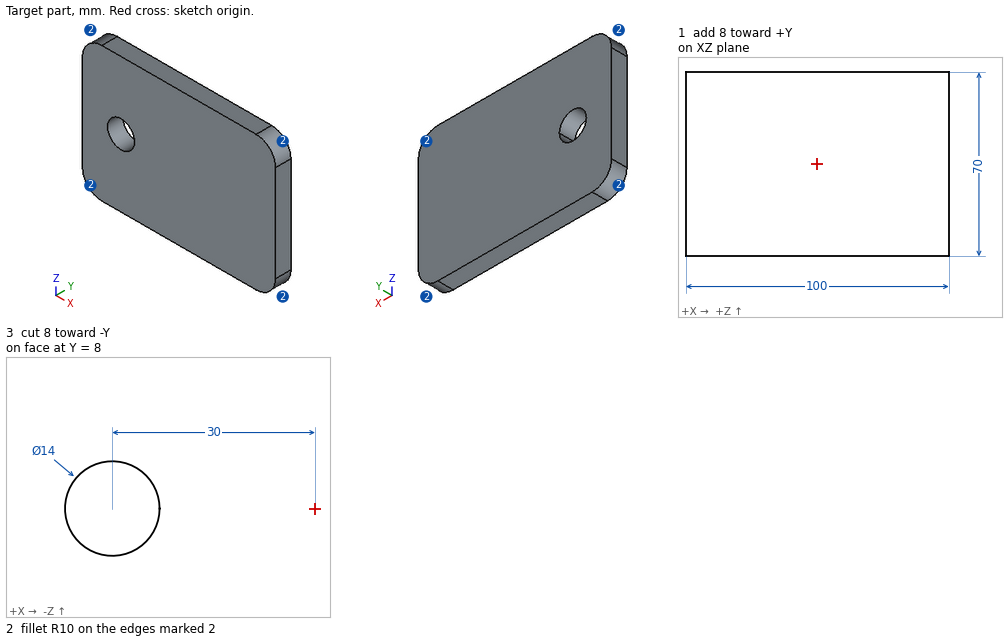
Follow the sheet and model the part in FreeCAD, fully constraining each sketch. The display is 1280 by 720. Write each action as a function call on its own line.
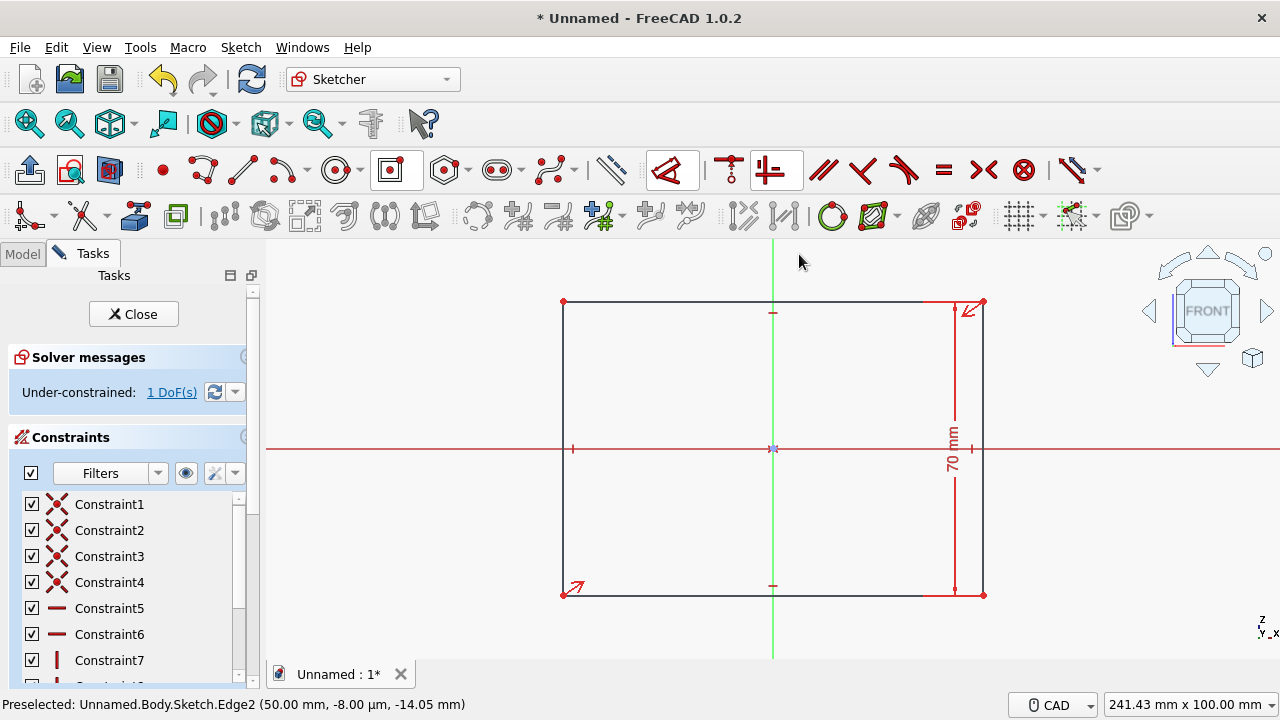
click(689, 596)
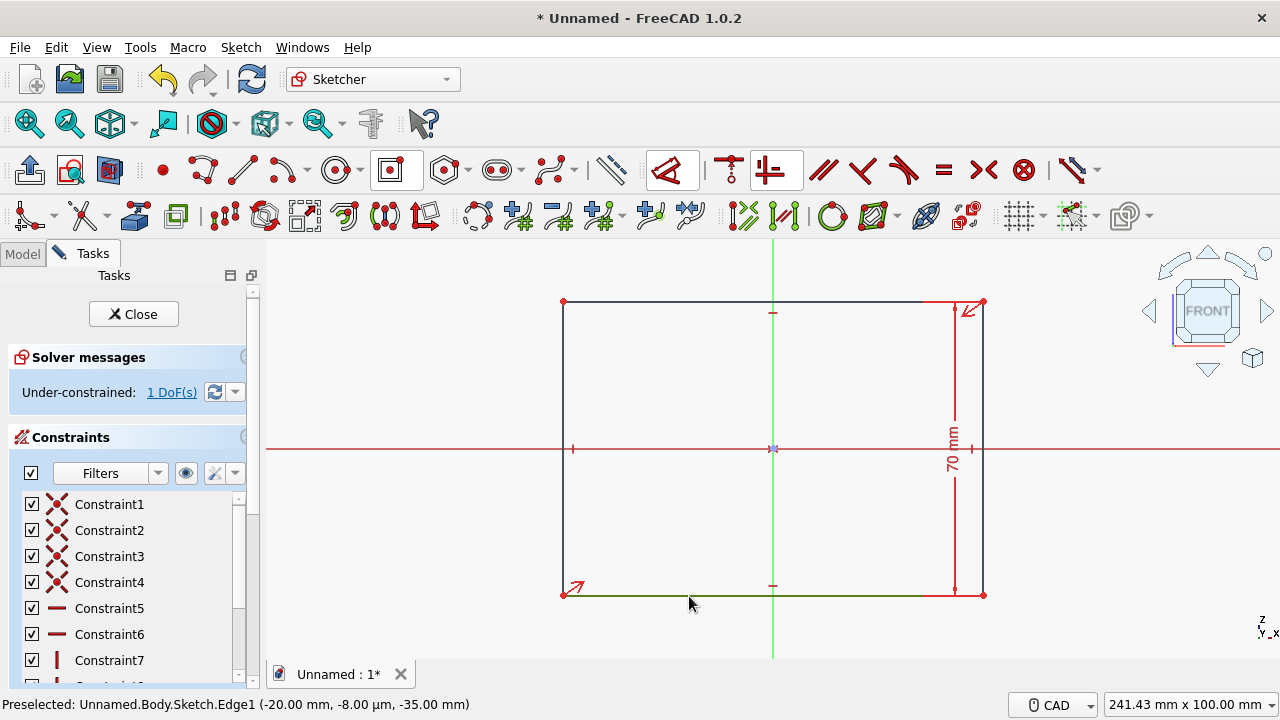
key(l)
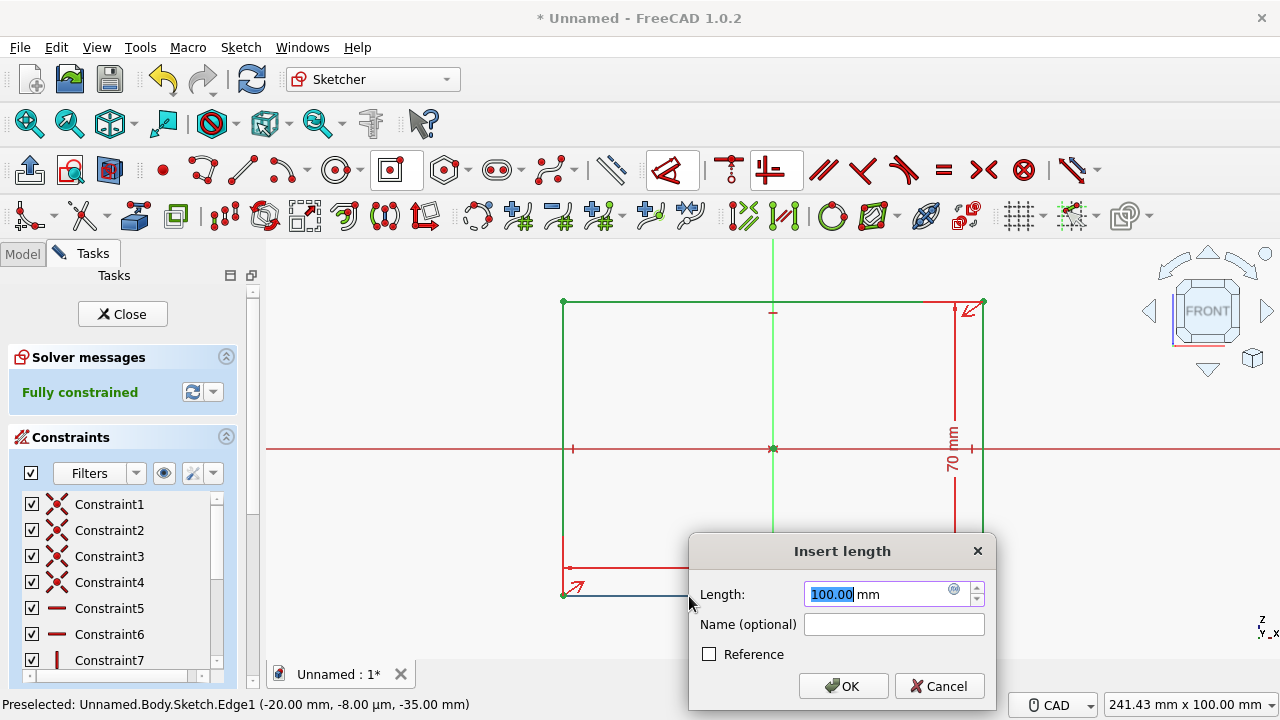
text(100)
key(Return)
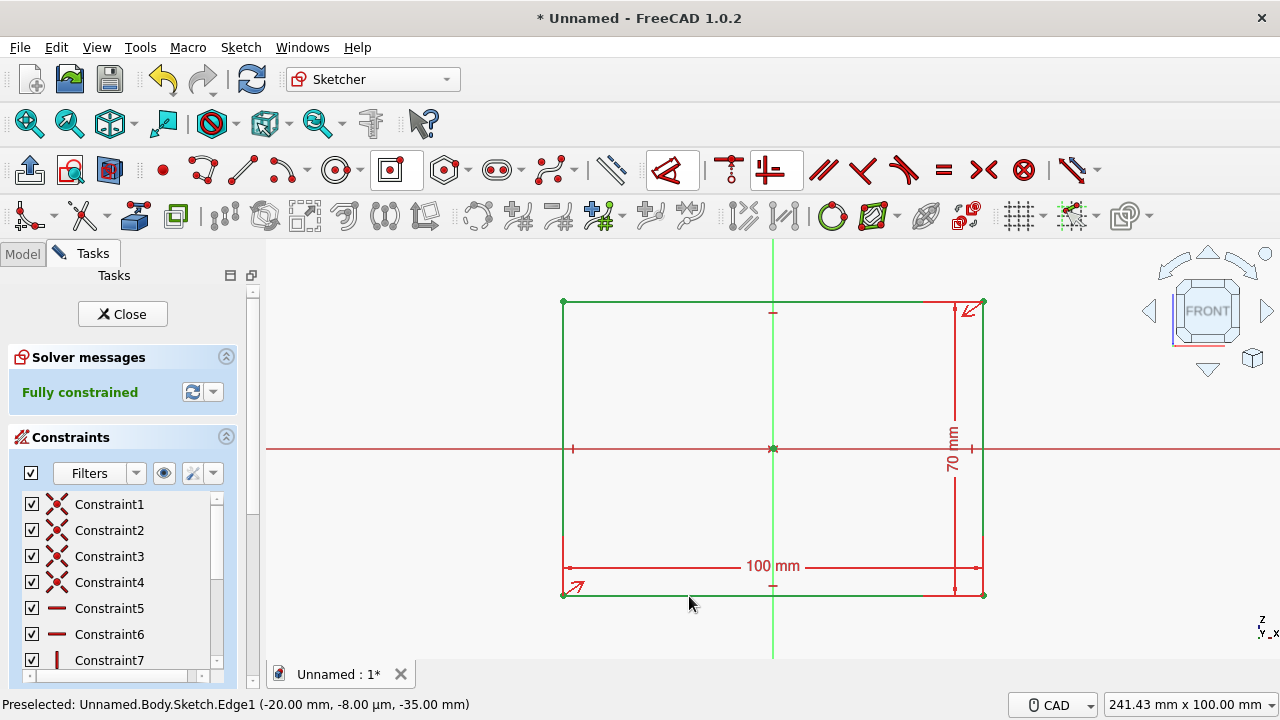
click(123, 314)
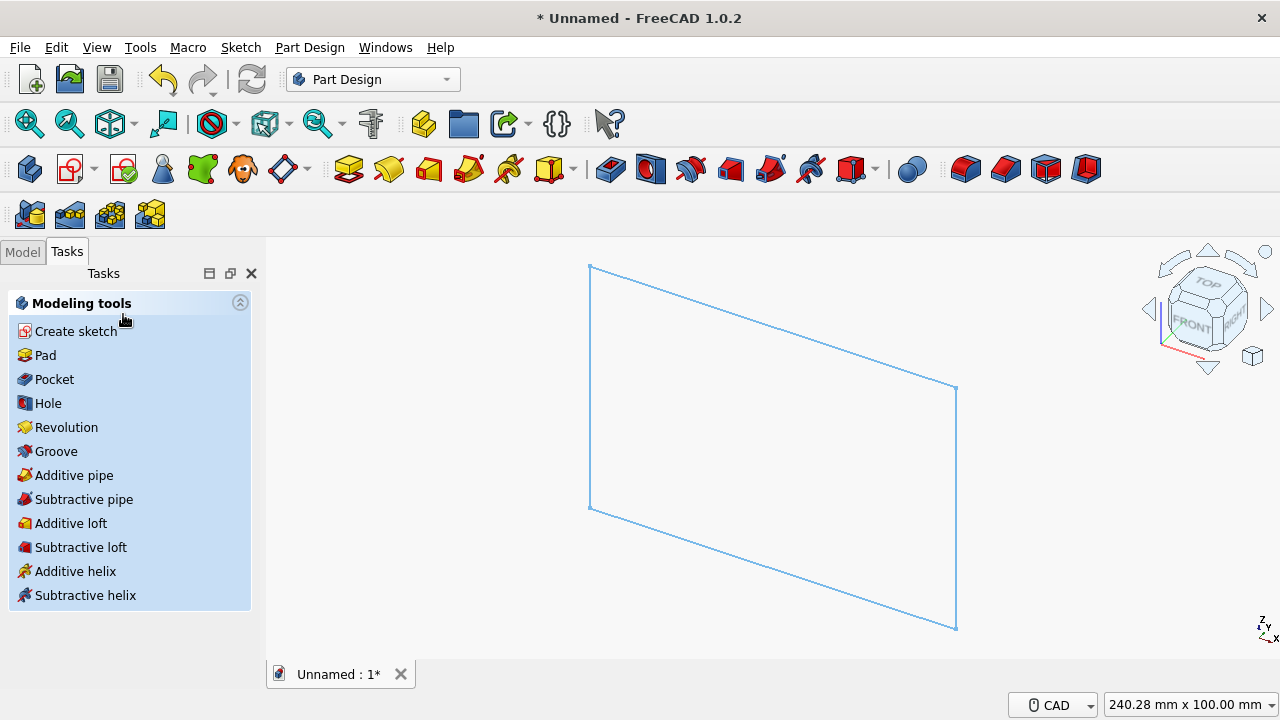
click(350, 170)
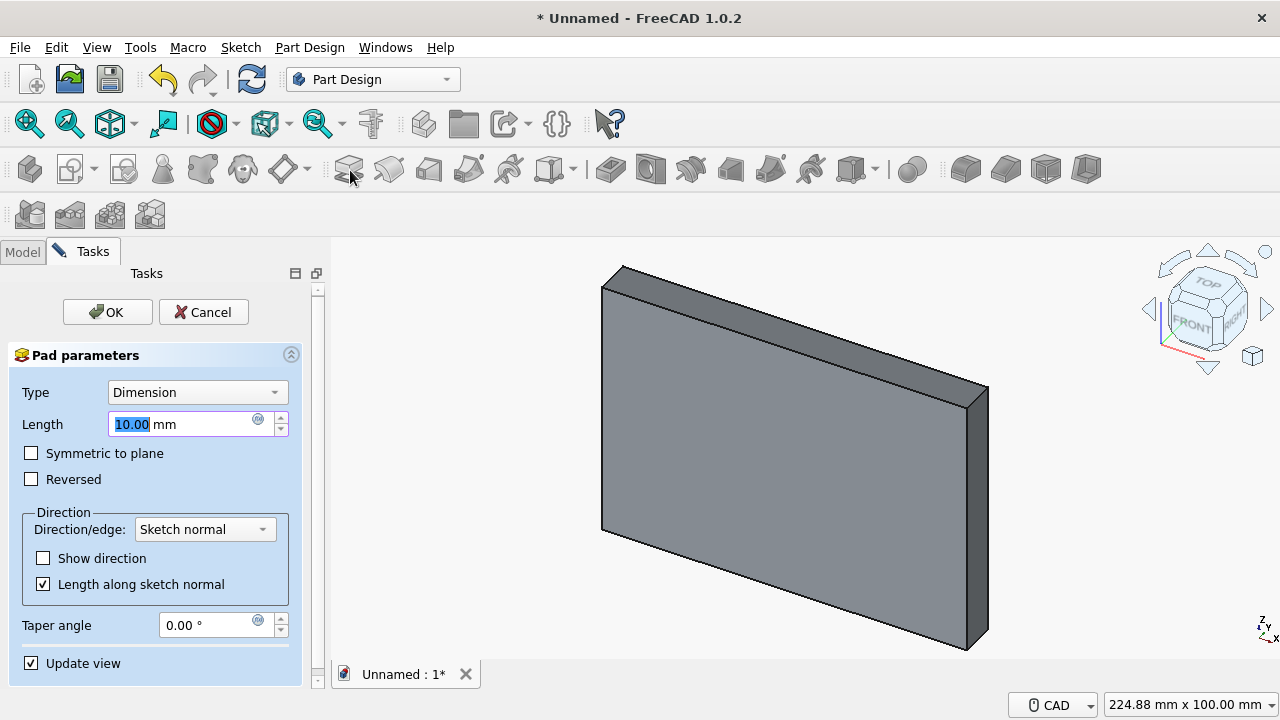
text(8)
key(Tab)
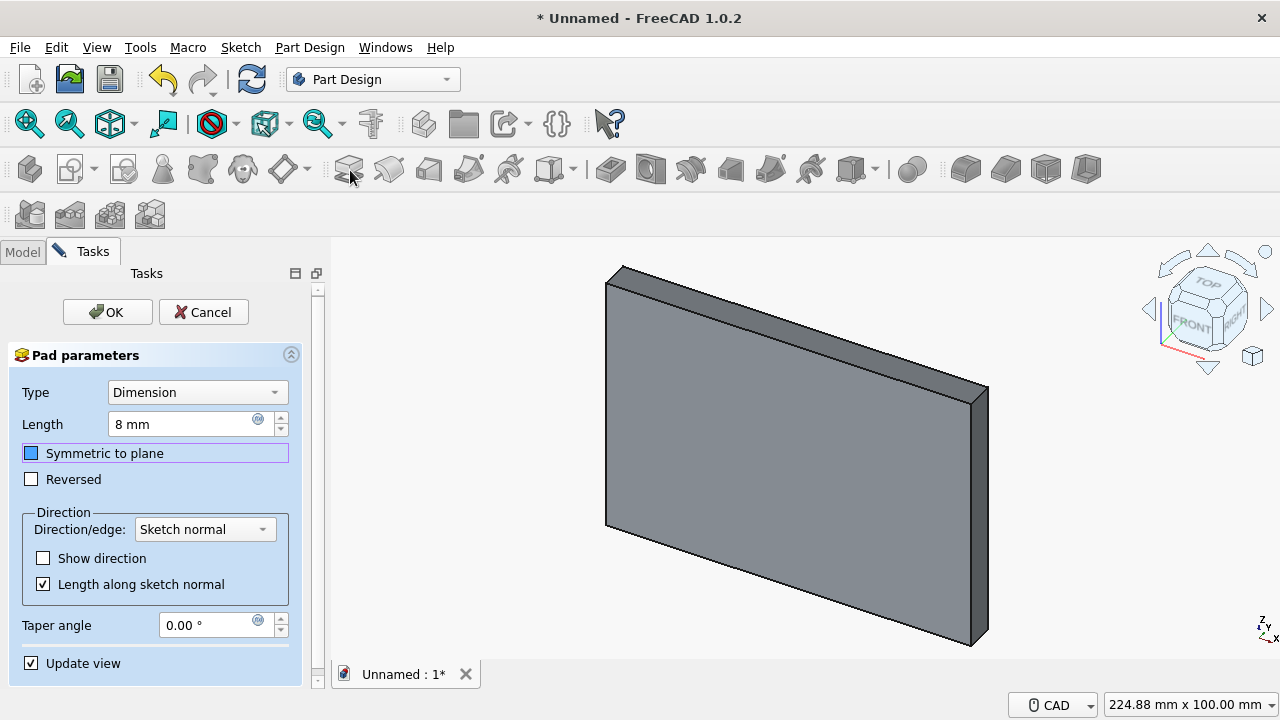
click(30, 479)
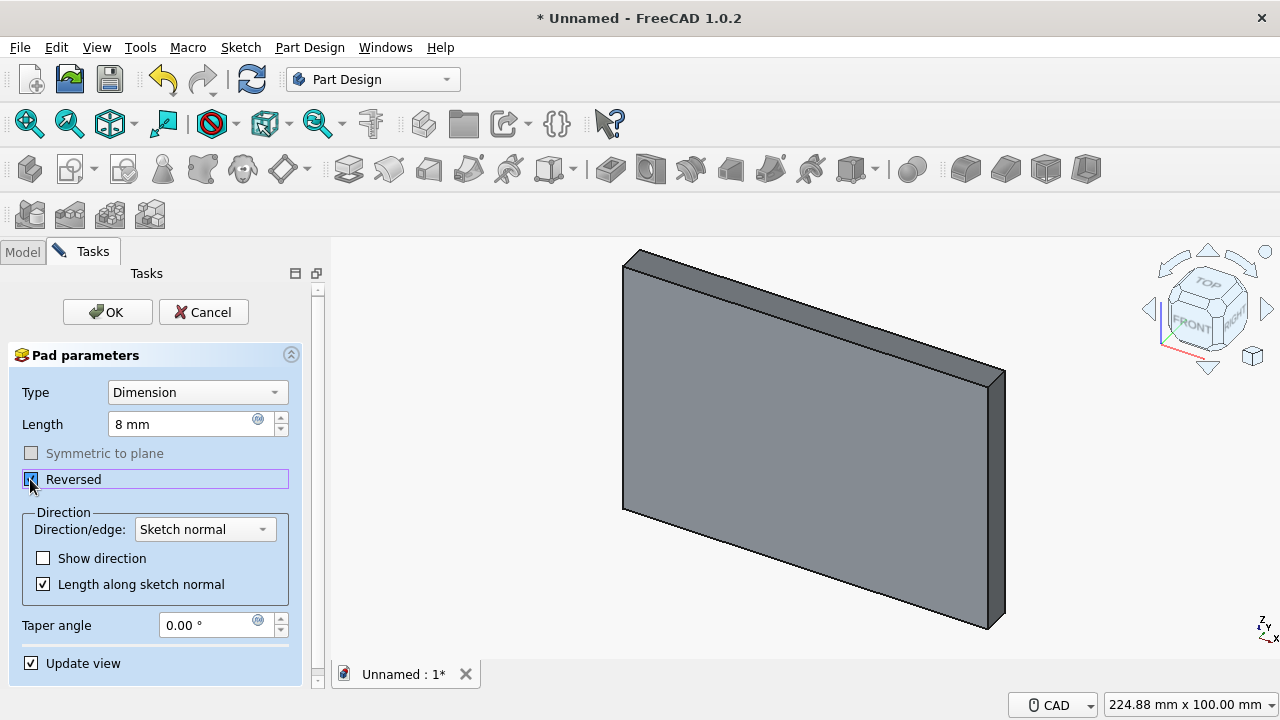
click(108, 312)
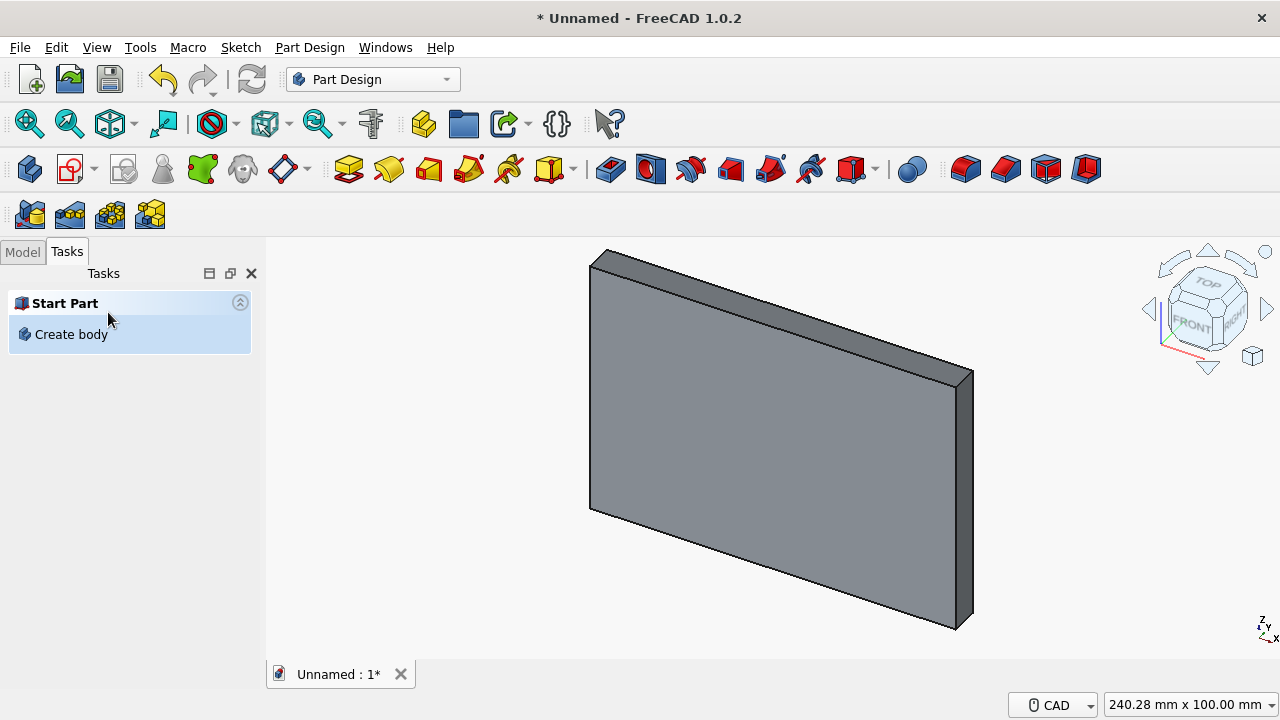
click(964, 378)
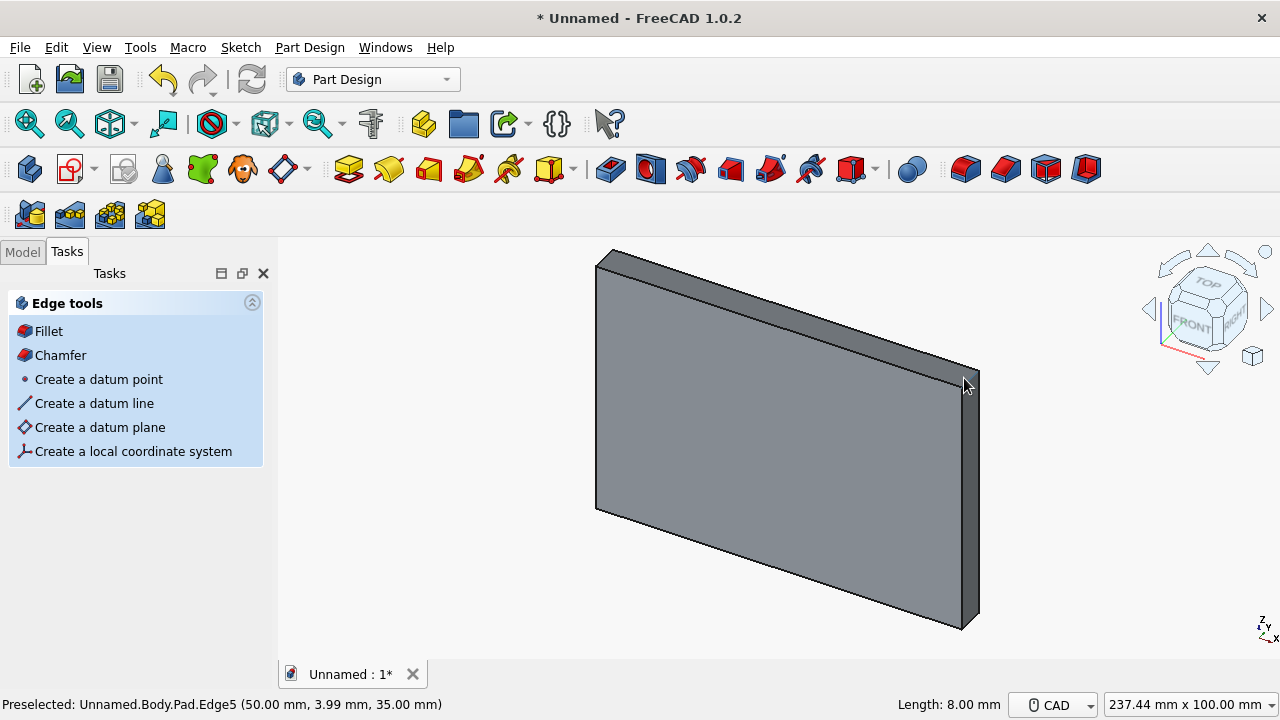
key(0)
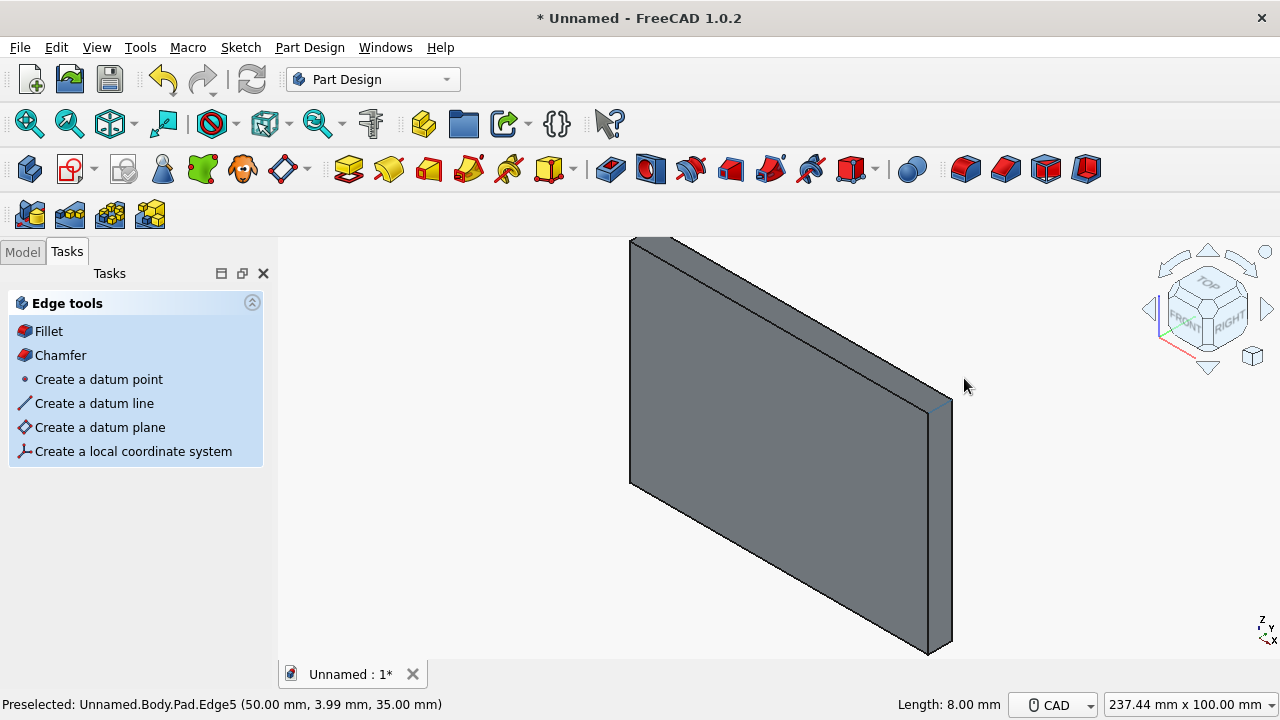
click(30, 124)